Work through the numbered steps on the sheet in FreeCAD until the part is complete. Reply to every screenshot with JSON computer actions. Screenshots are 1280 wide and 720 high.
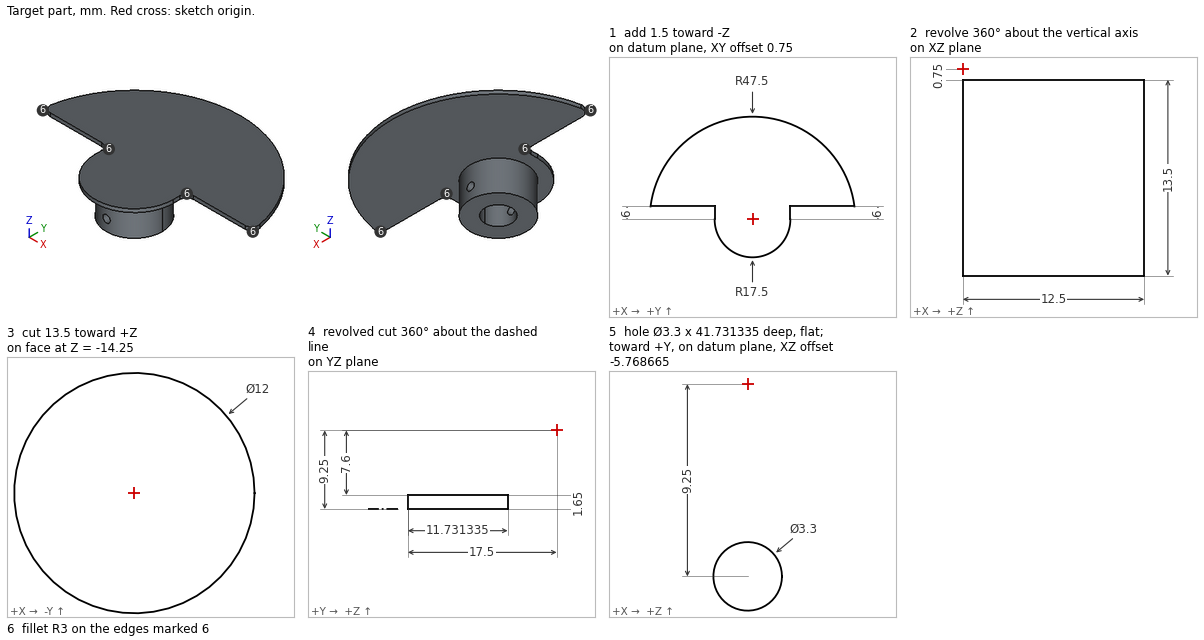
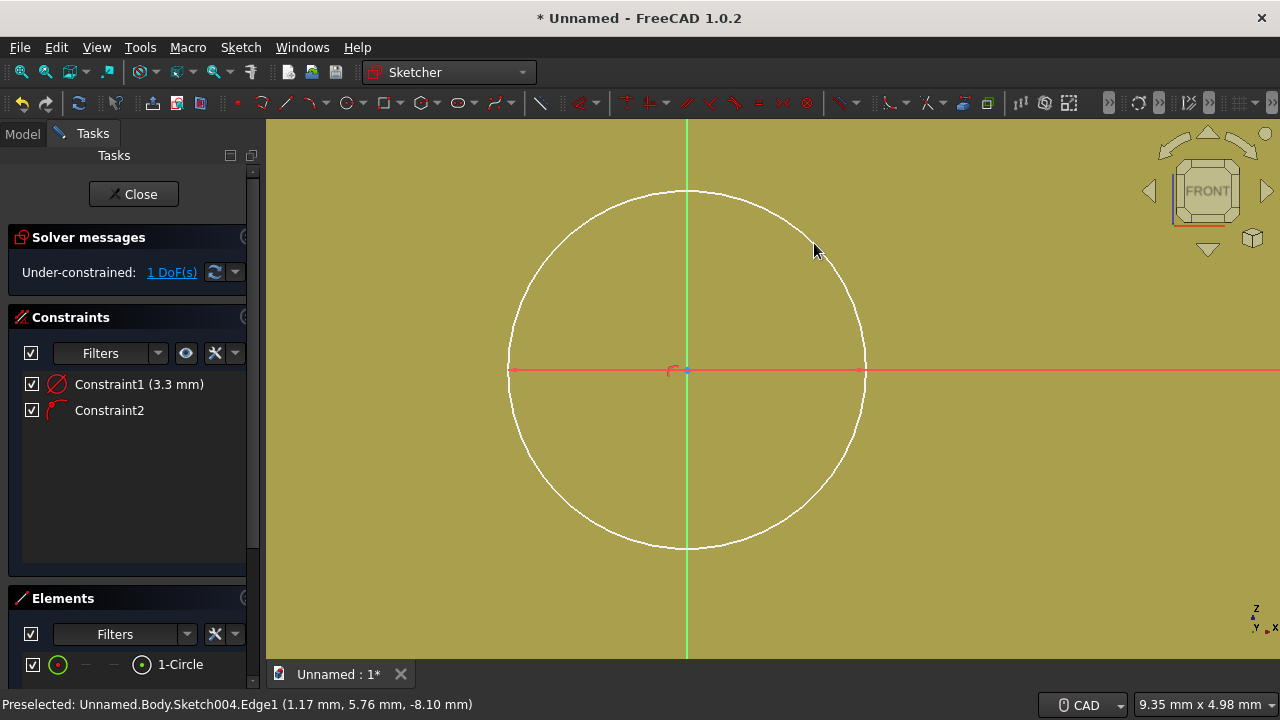
{"action": "key", "text": "d"}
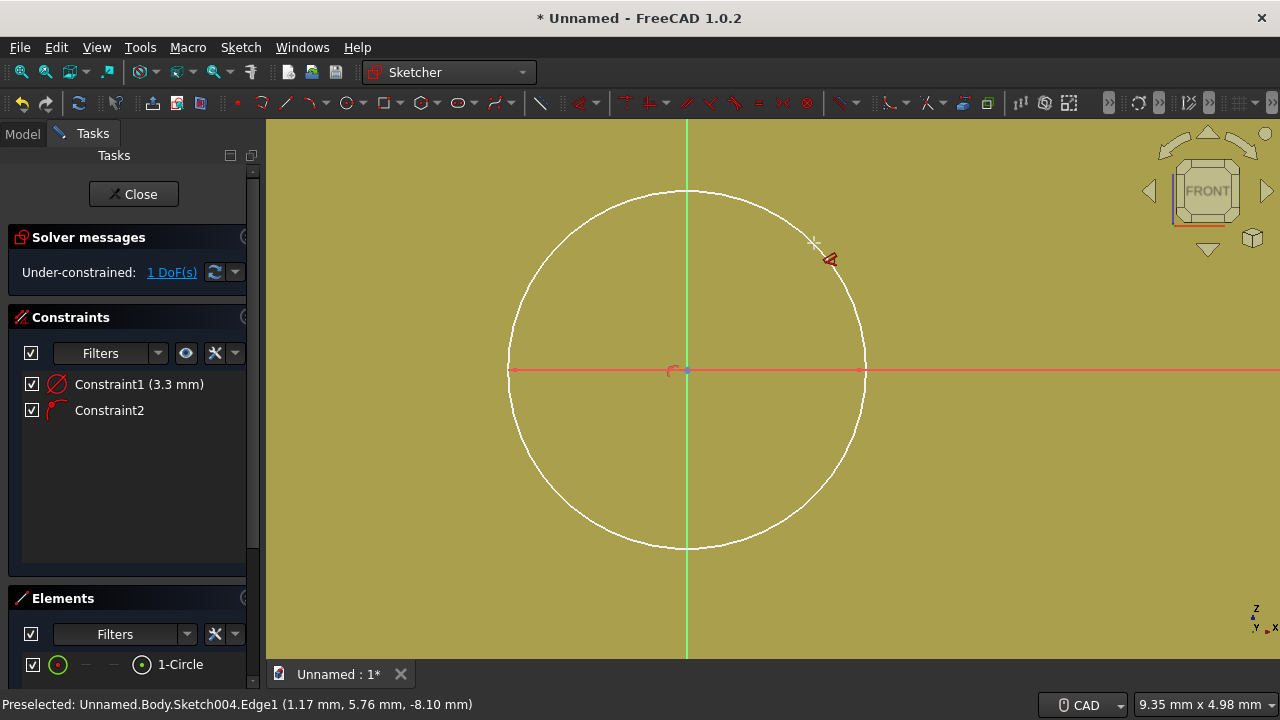
{"action": "left_click", "coordinate": [687, 370]}
{"action": "left_click", "coordinate": [721, 259]}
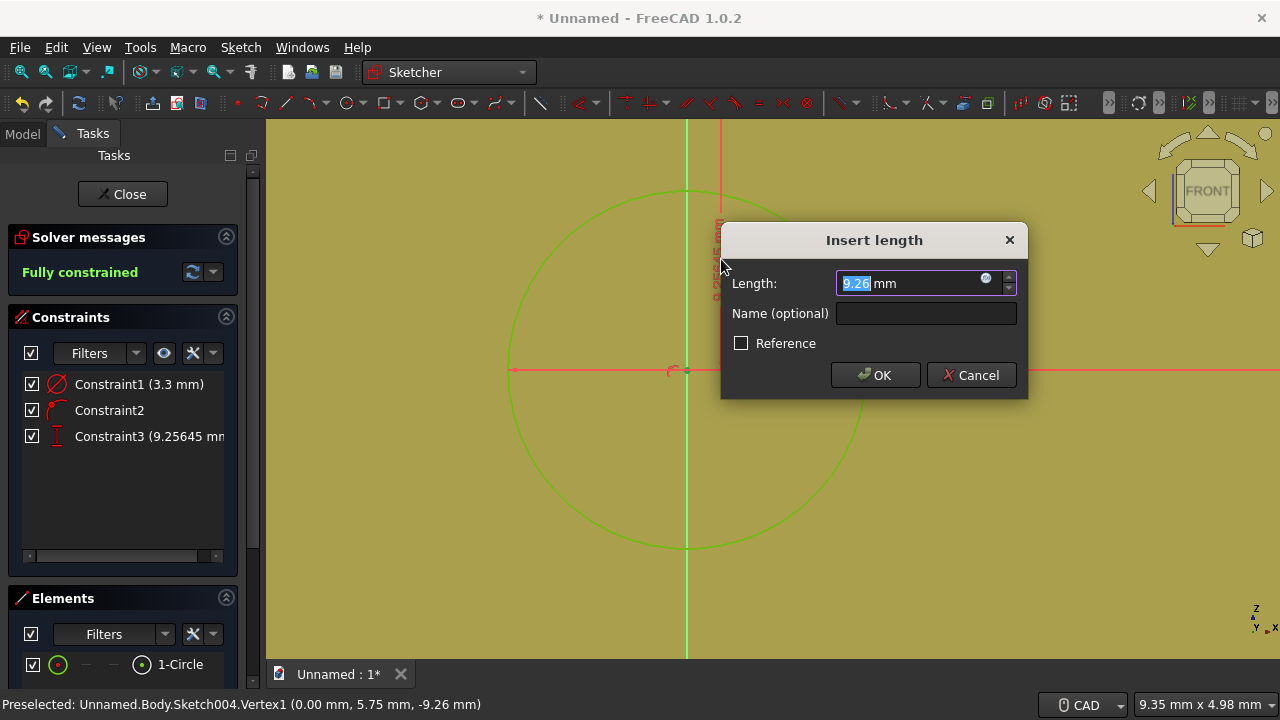
{"action": "type", "text": "9.25"}
{"action": "key", "text": "Return"}
{"action": "key", "text": "Escape"}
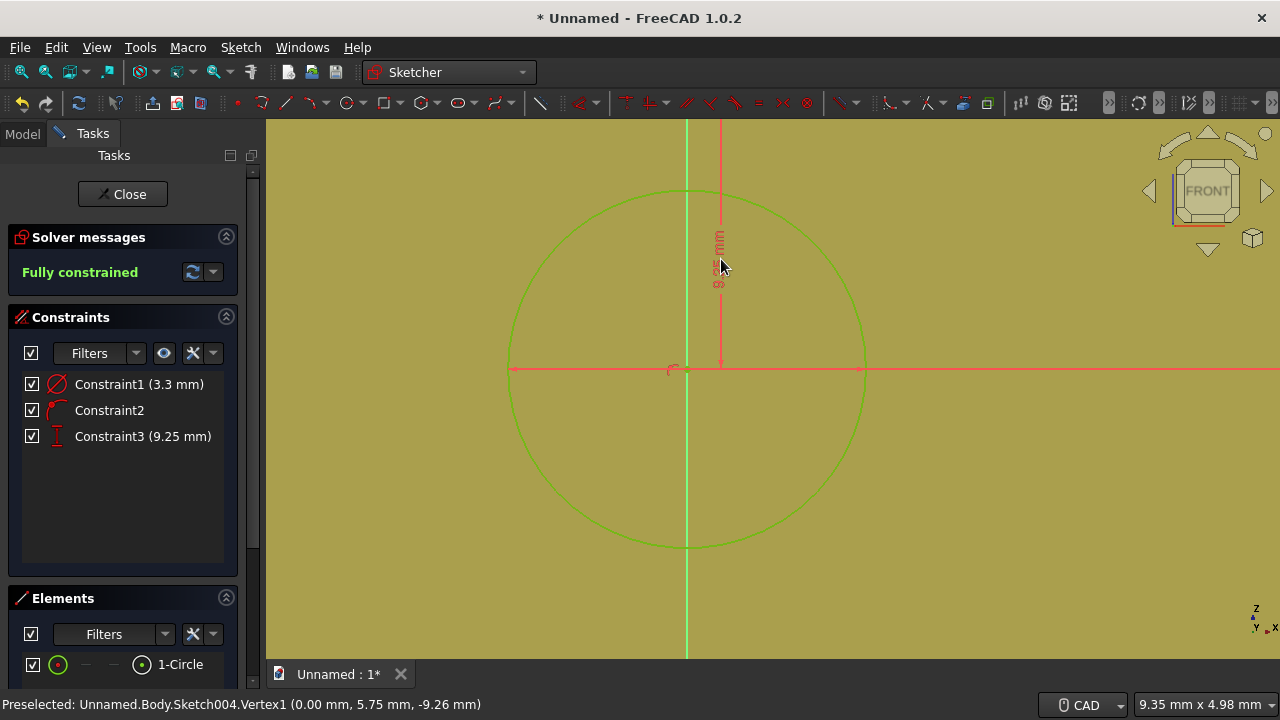
{"action": "left_click", "coordinate": [123, 194]}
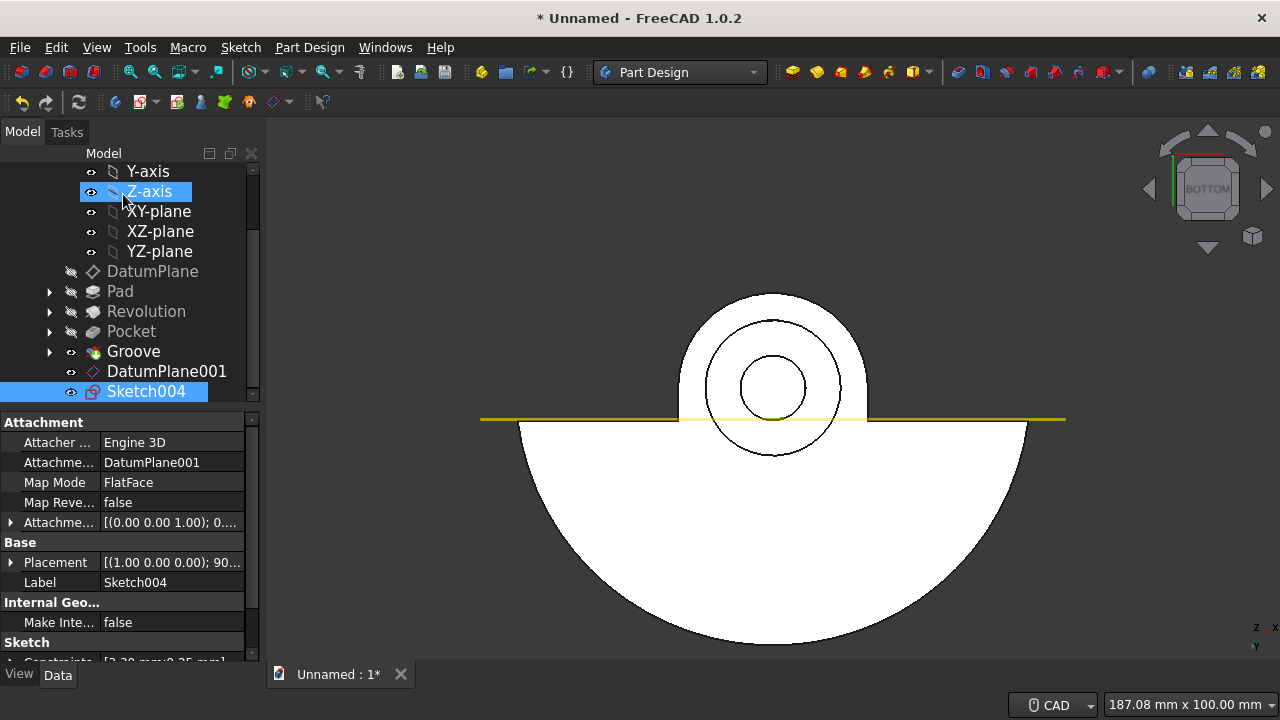
{"action": "left_click", "coordinate": [984, 72]}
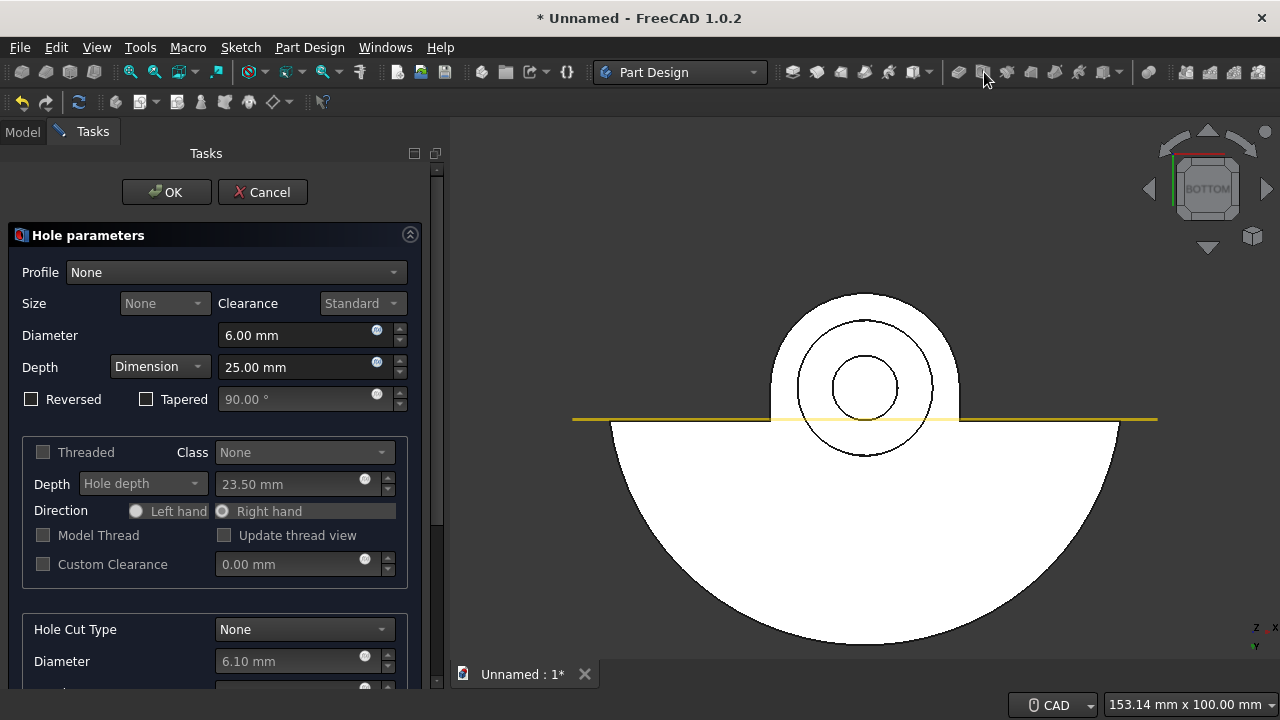
{"action": "triple_click", "coordinate": [305, 335]}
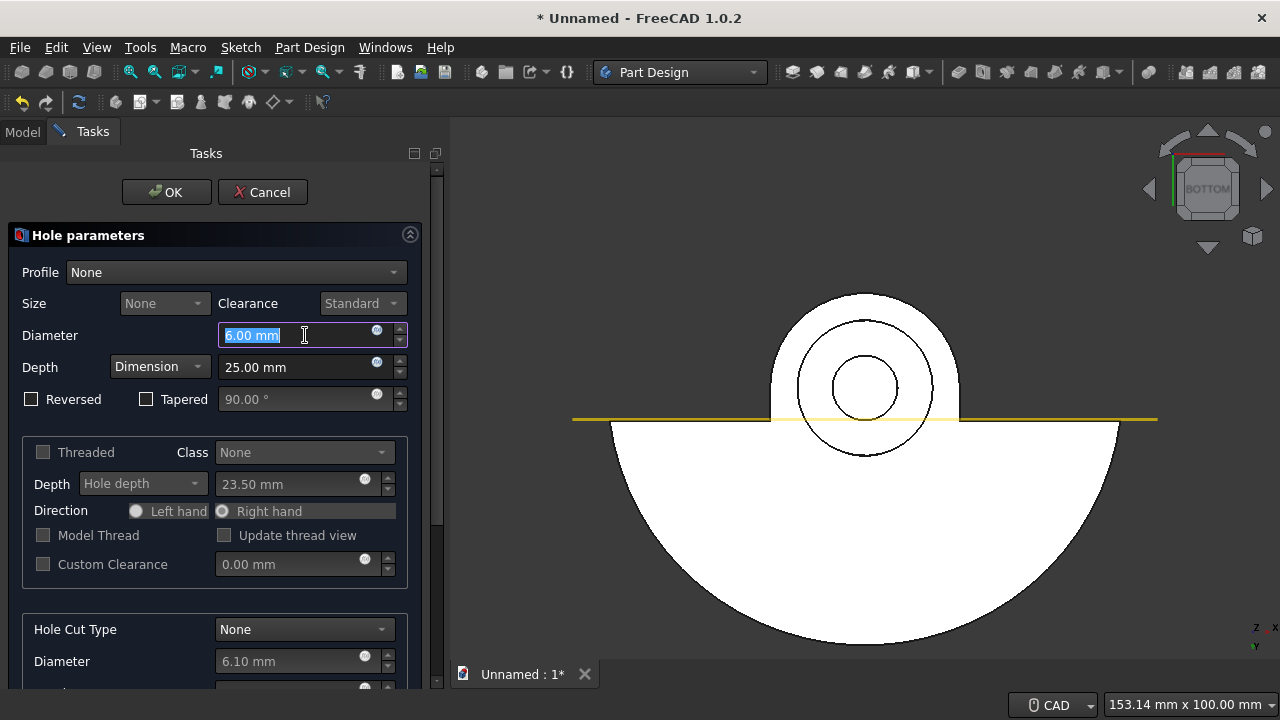
{"action": "type", "text": "3.3"}
{"action": "key", "text": "Tab"}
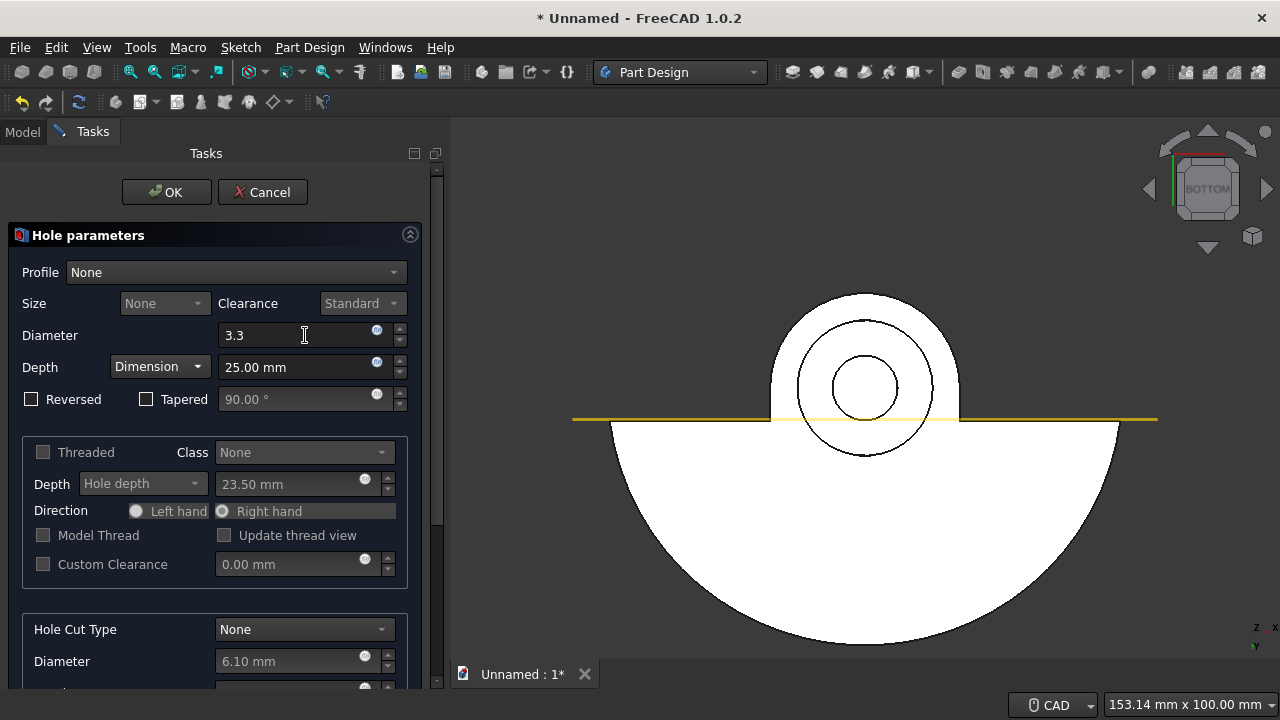
{"action": "triple_click", "coordinate": [305, 367]}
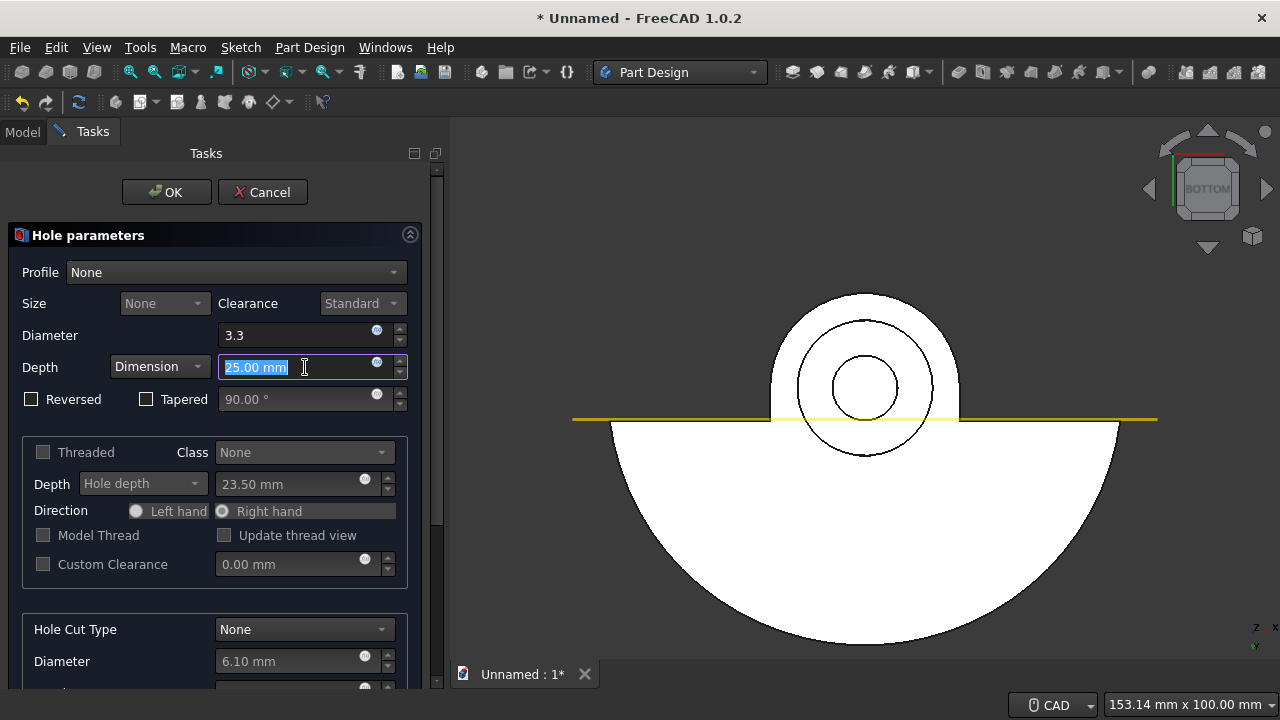
{"action": "type", "text": "41.731335"}
{"action": "key", "text": "Tab"}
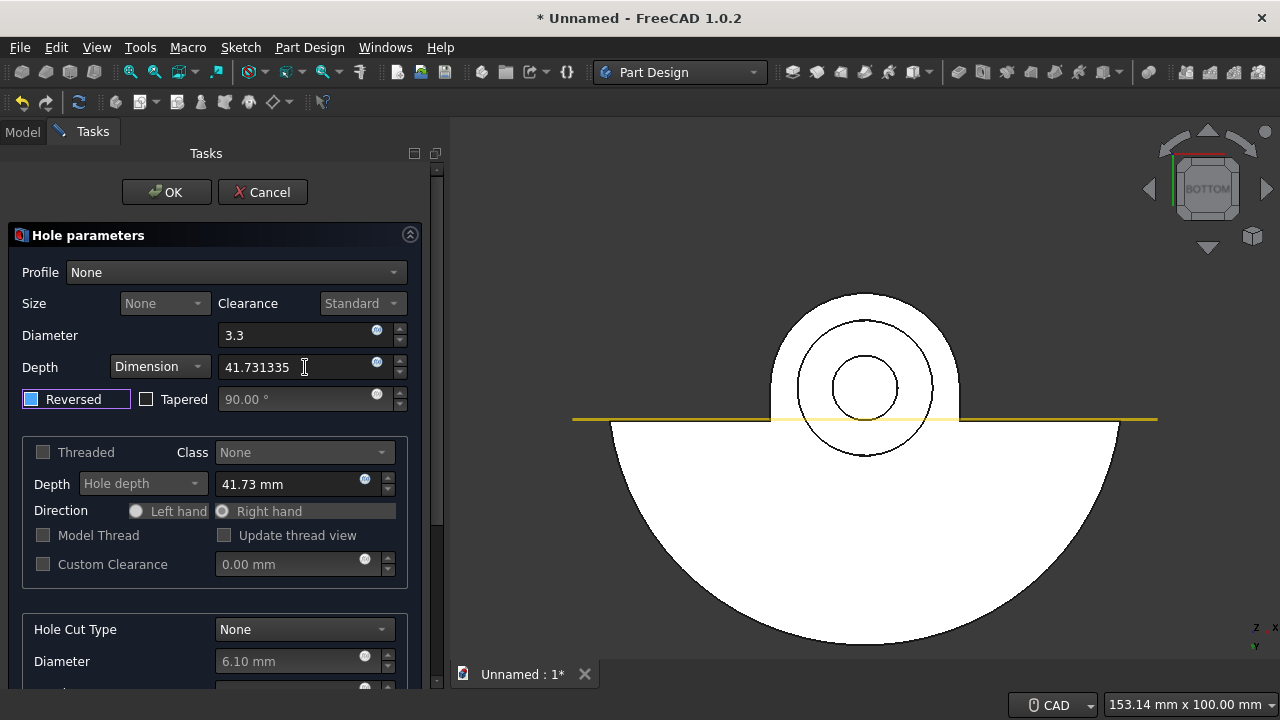
{"action": "scroll", "coordinate": [437, 426], "scroll_direction": "down", "scroll_amount": 4}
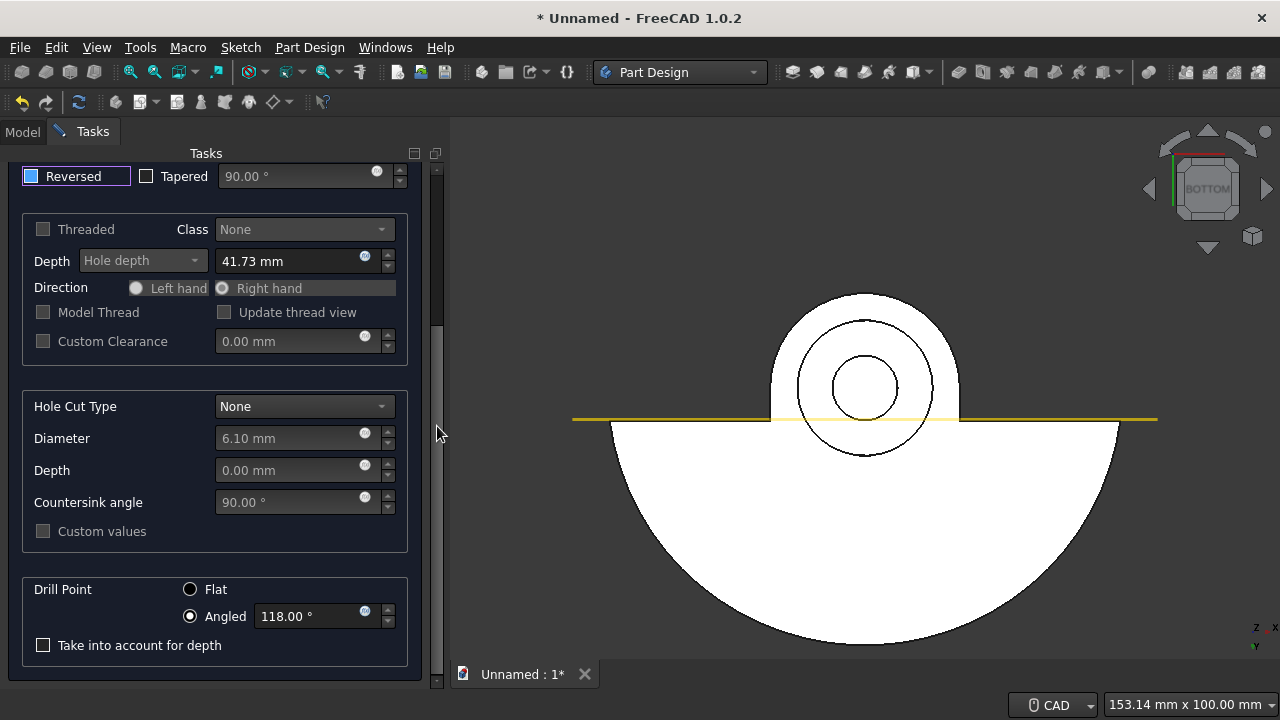
{"action": "left_click", "coordinate": [191, 589]}